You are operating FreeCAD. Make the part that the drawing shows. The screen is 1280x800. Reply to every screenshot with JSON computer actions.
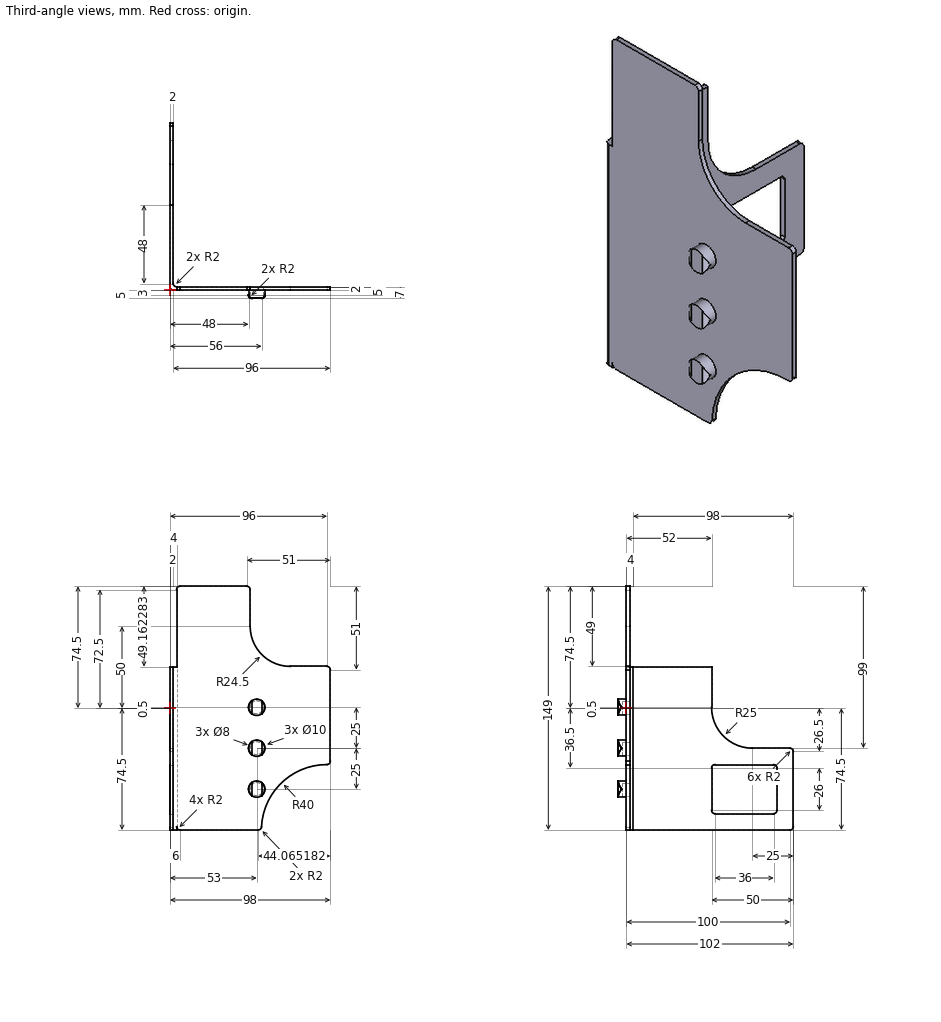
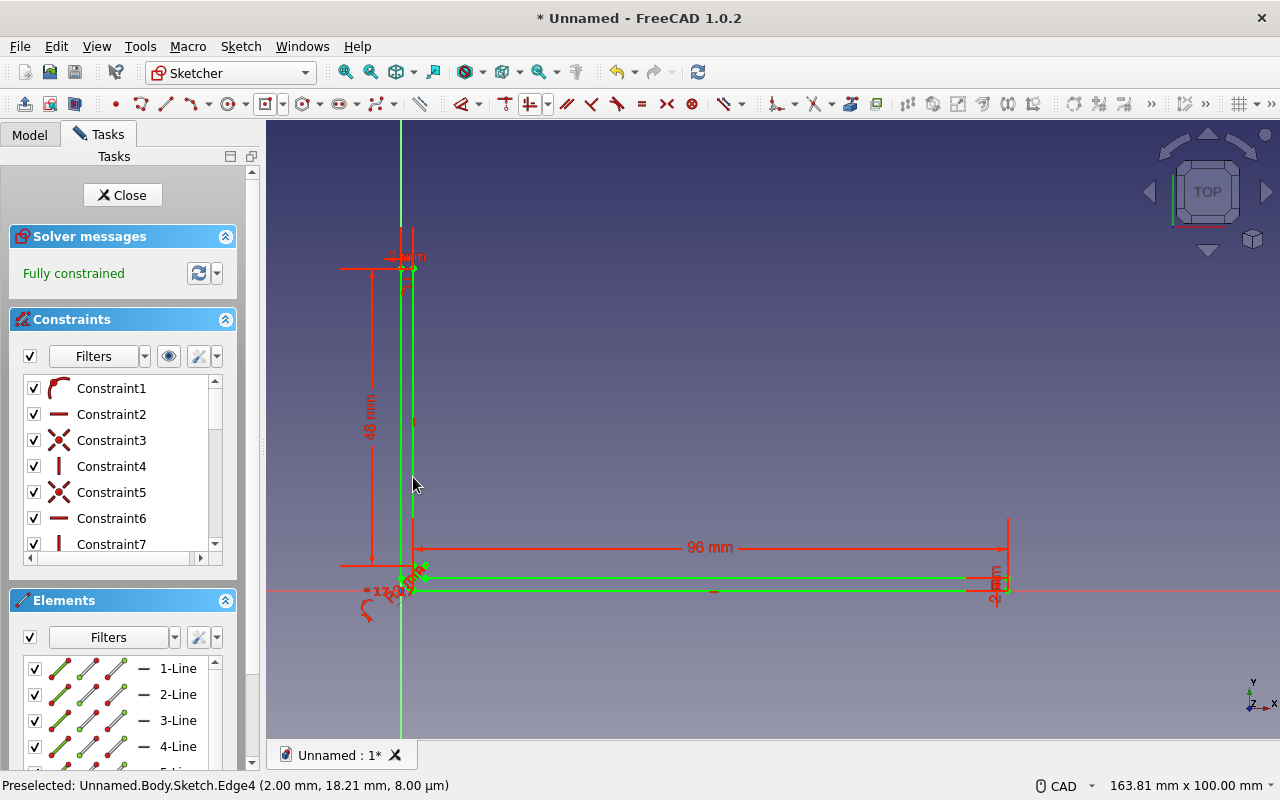
{"action": "left_click", "coordinate": [123, 195]}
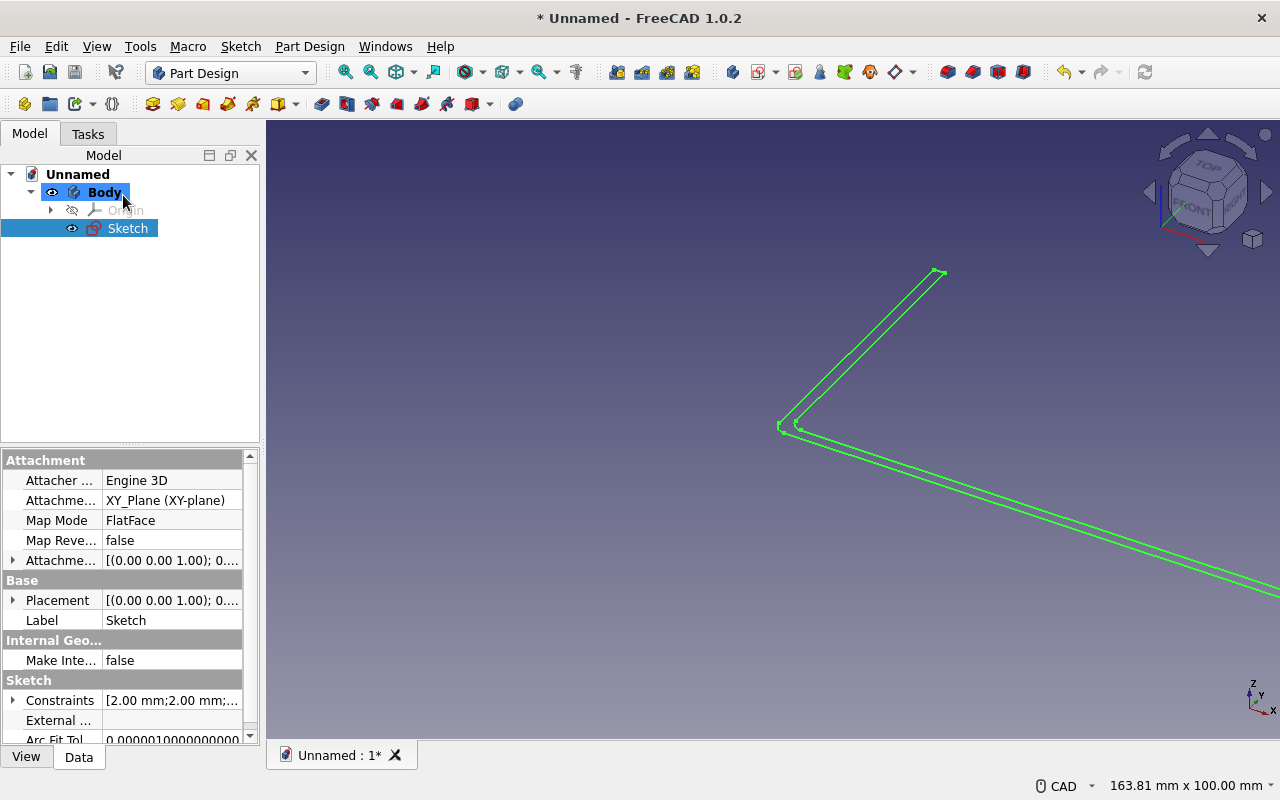
{"action": "left_click", "coordinate": [153, 104]}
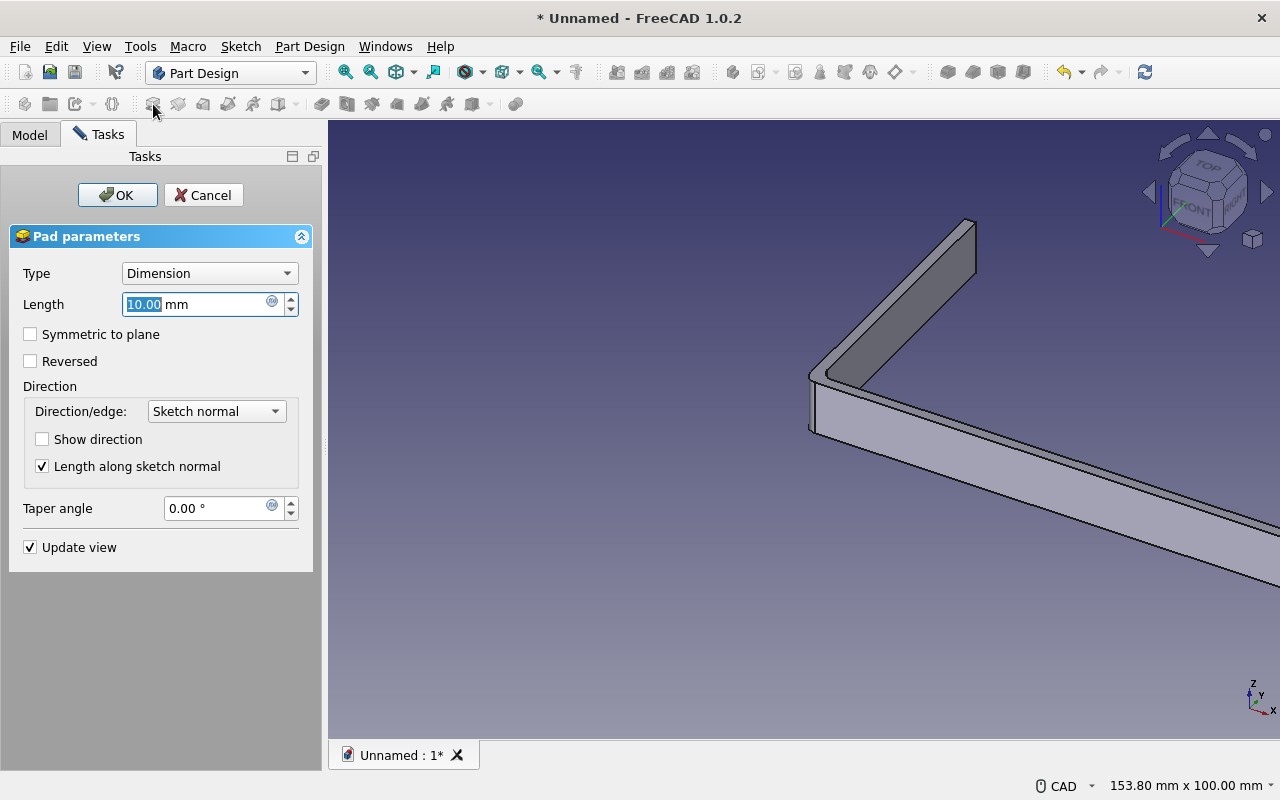
{"action": "type", "text": "149"}
{"action": "key", "text": "Tab"}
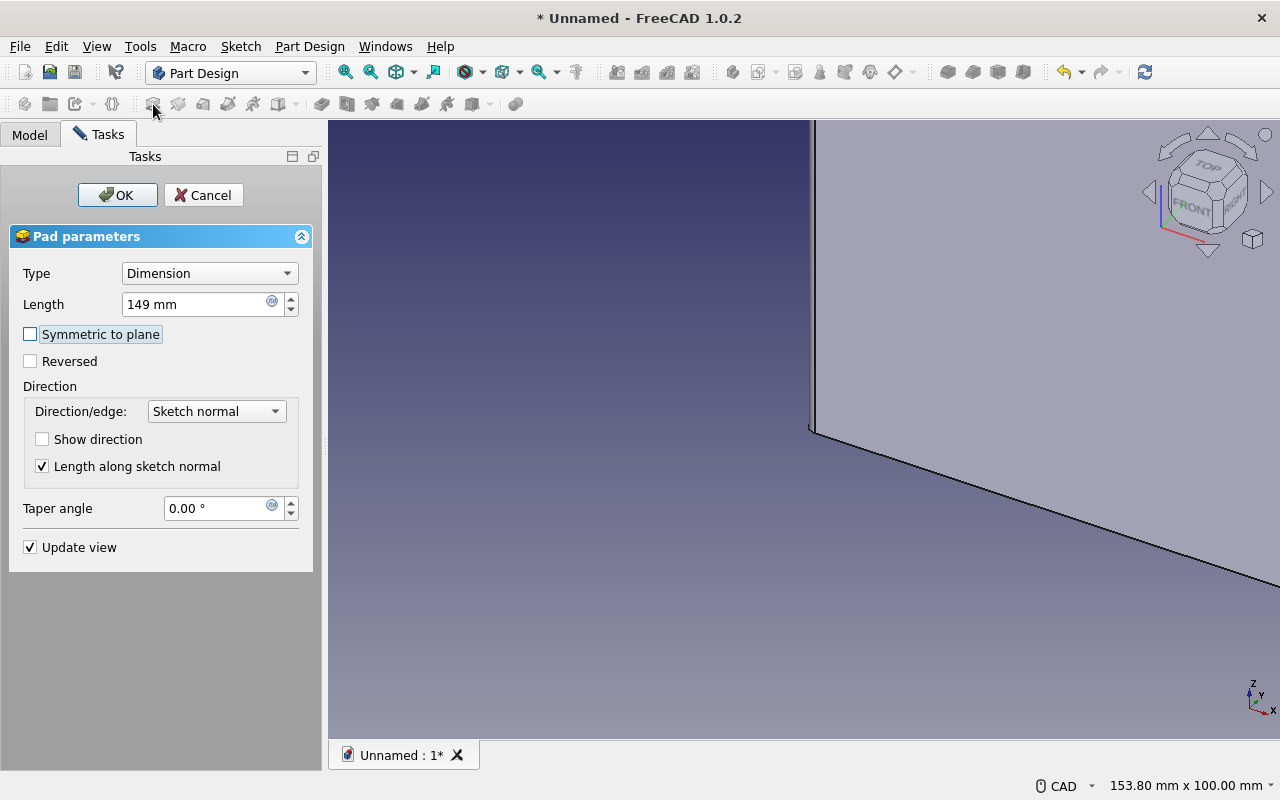
{"action": "left_click", "coordinate": [31, 334]}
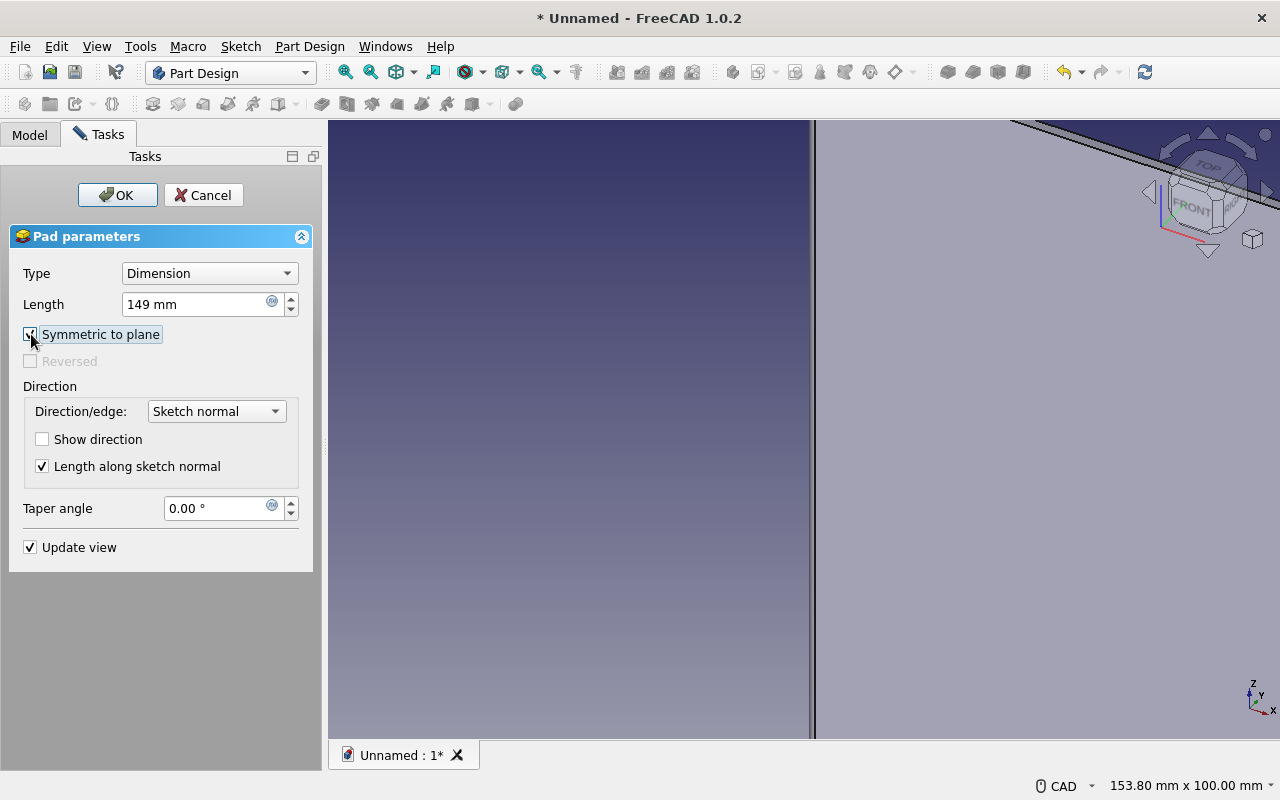
{"action": "left_click", "coordinate": [118, 195]}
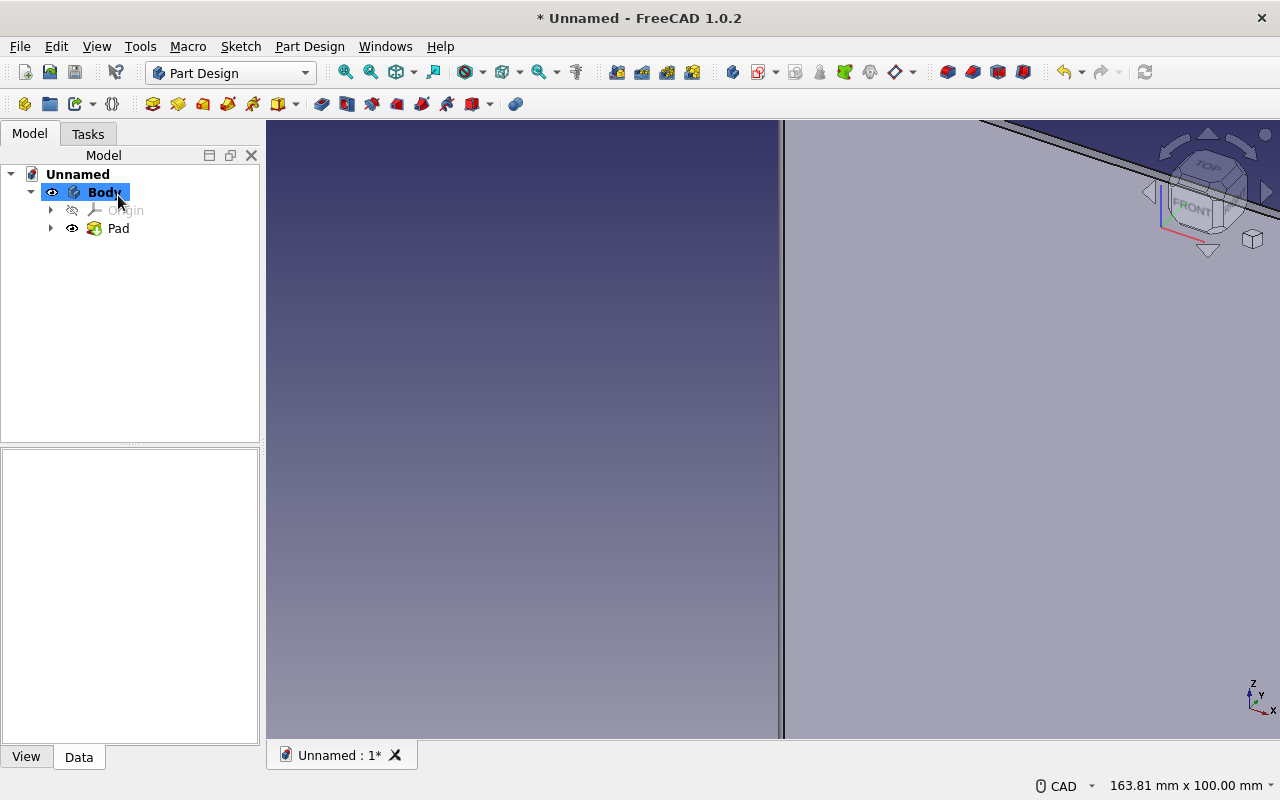
{"action": "key", "text": "v f"}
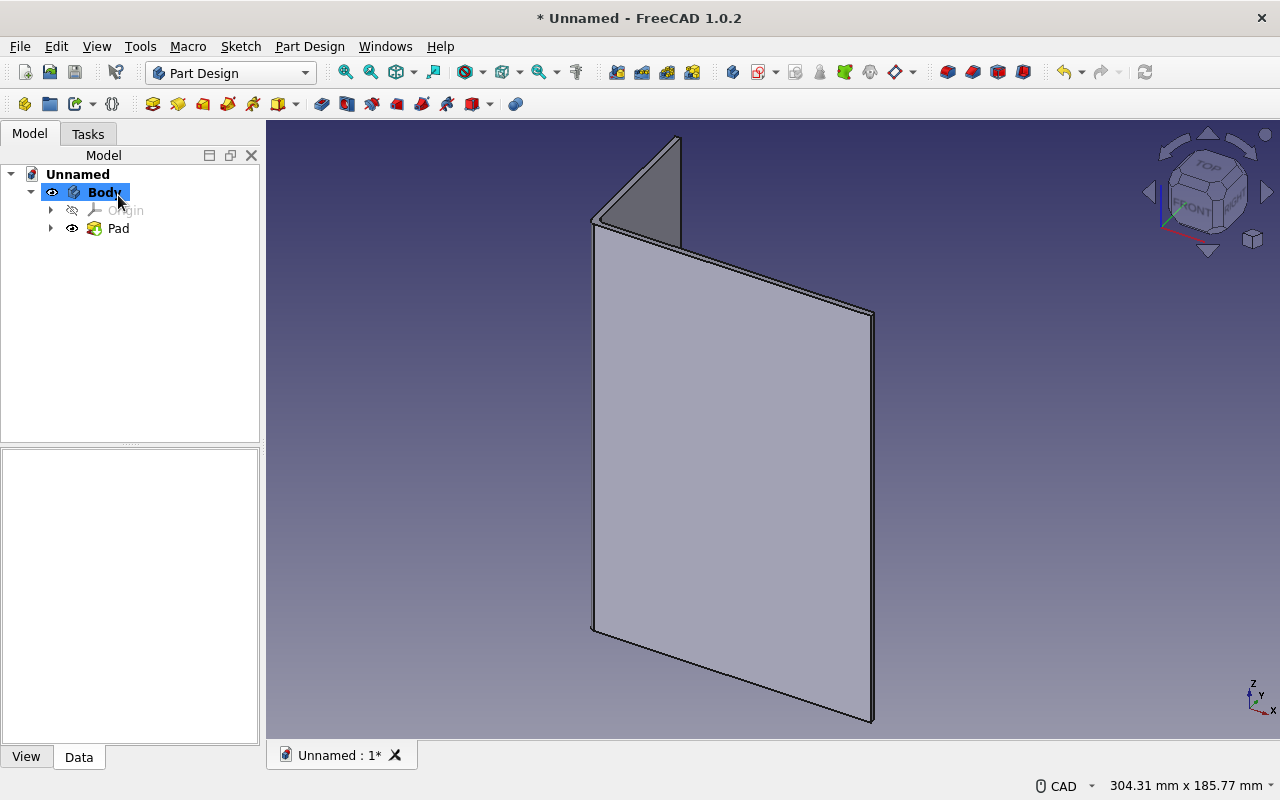
{"action": "key", "text": "0"}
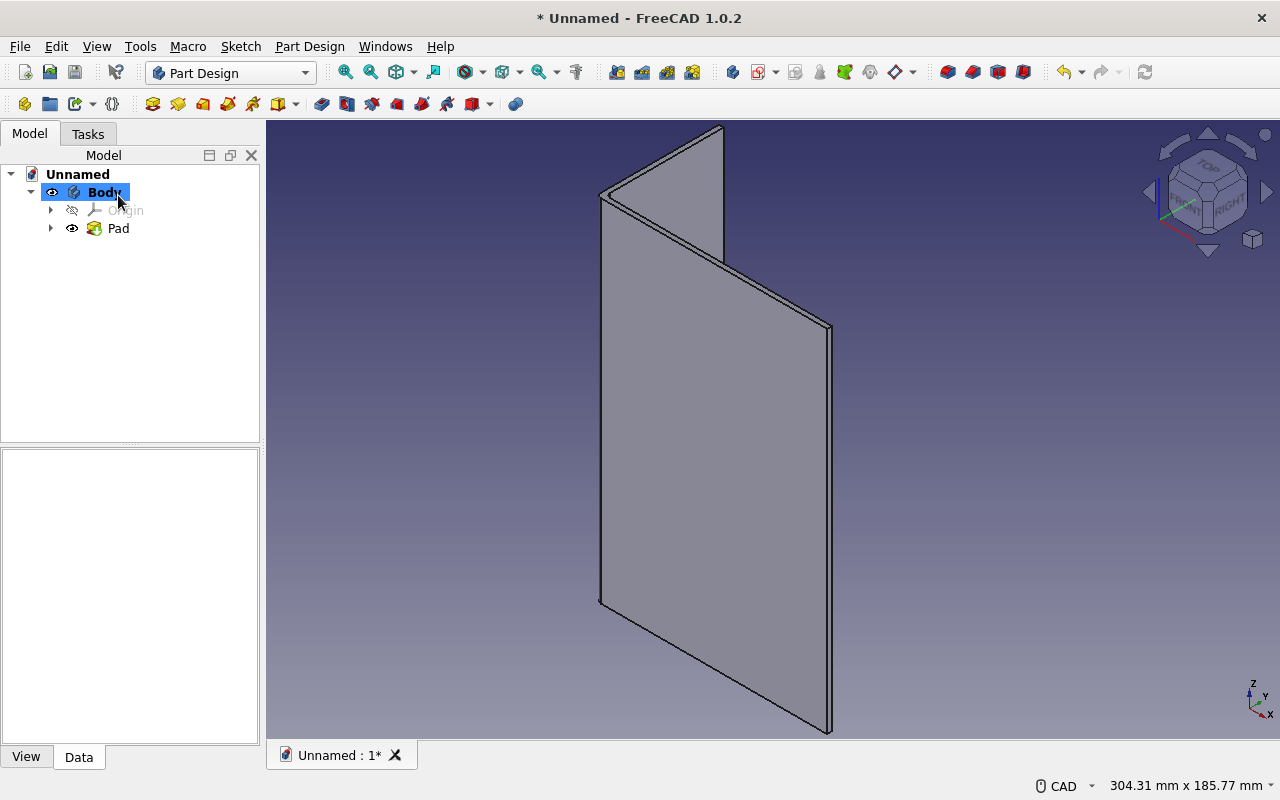
{"action": "key", "text": "3"}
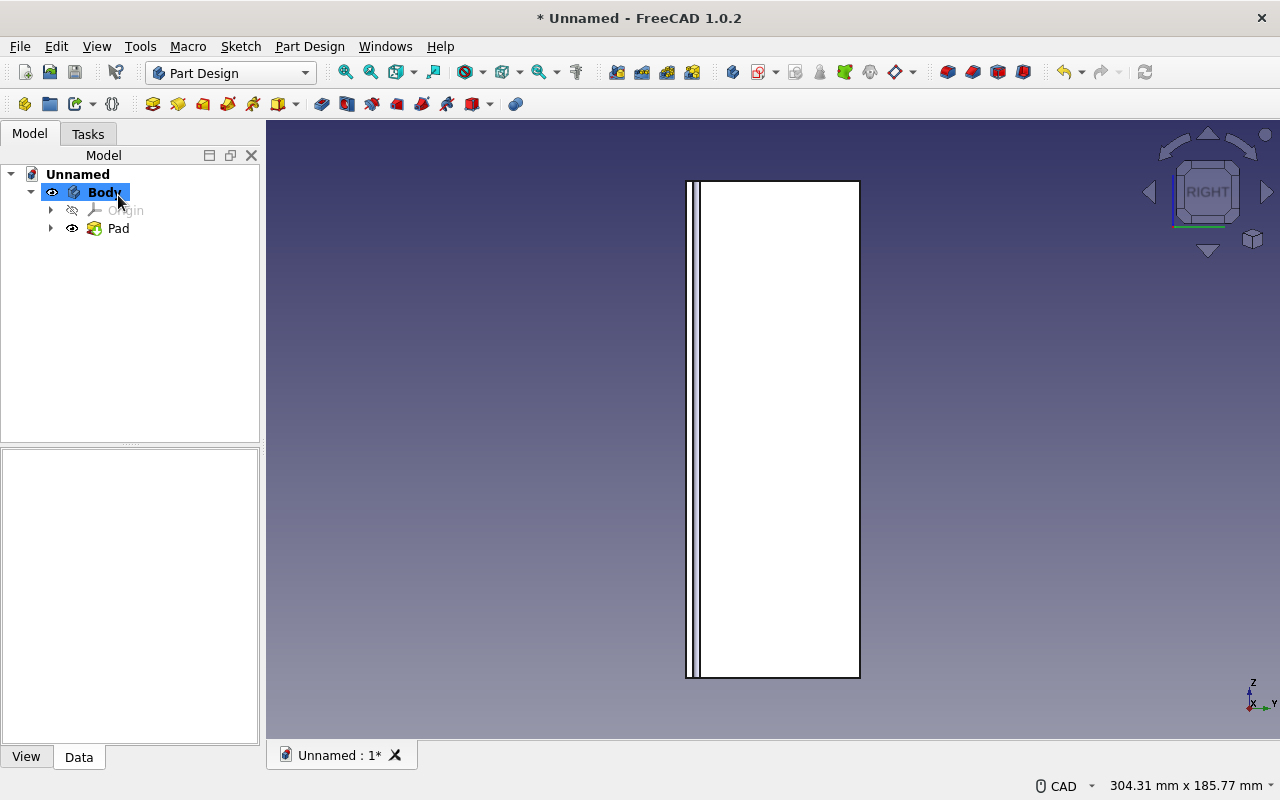
{"action": "left_click", "coordinate": [780, 287]}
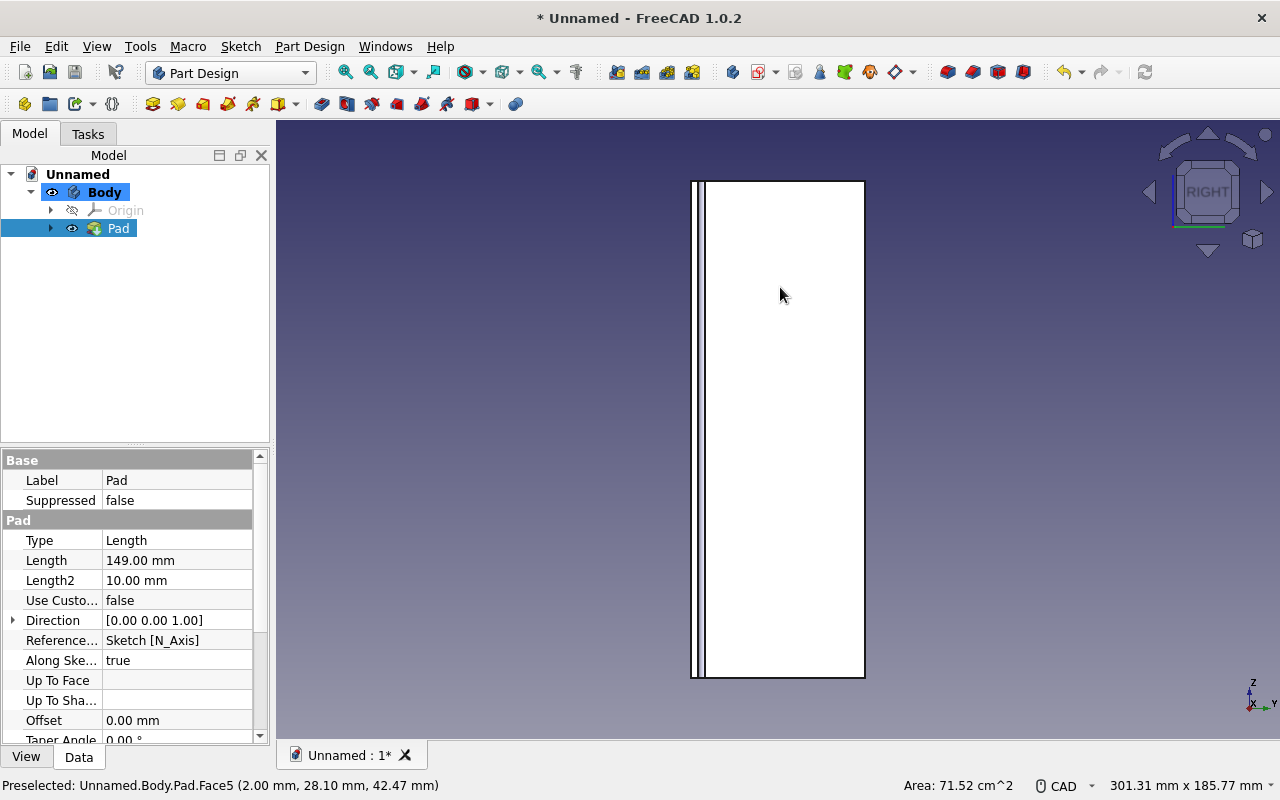
{"action": "left_click", "coordinate": [758, 72]}